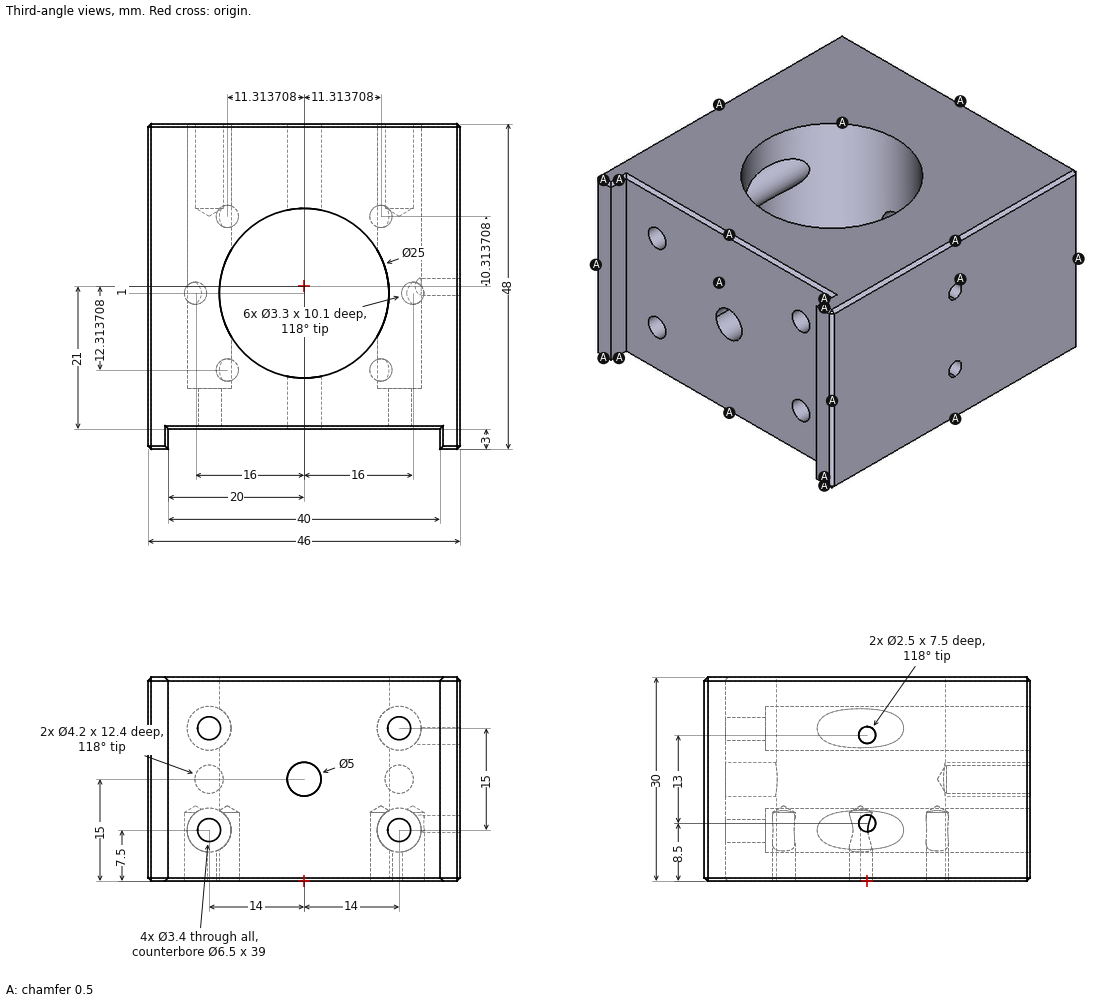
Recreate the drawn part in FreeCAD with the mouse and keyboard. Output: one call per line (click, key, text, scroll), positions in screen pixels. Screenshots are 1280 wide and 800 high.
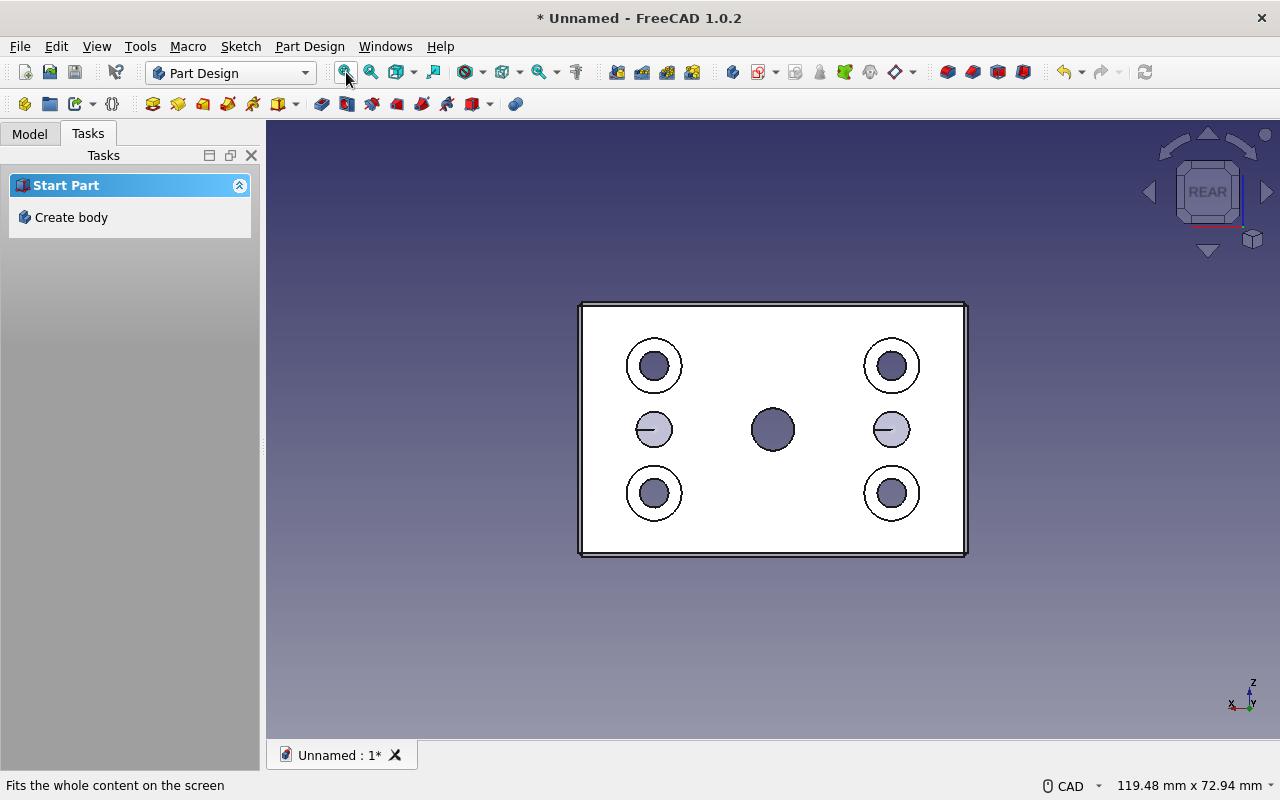
key(0)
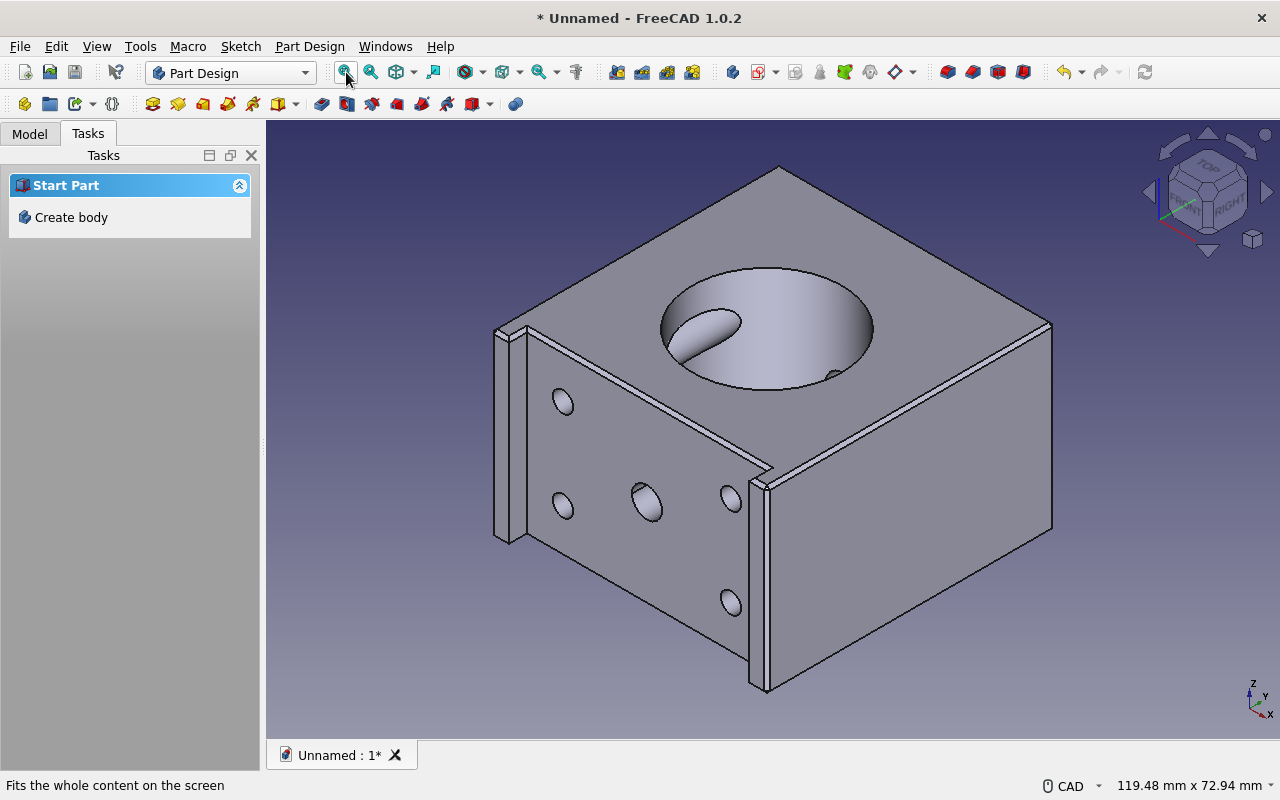
click(951, 485)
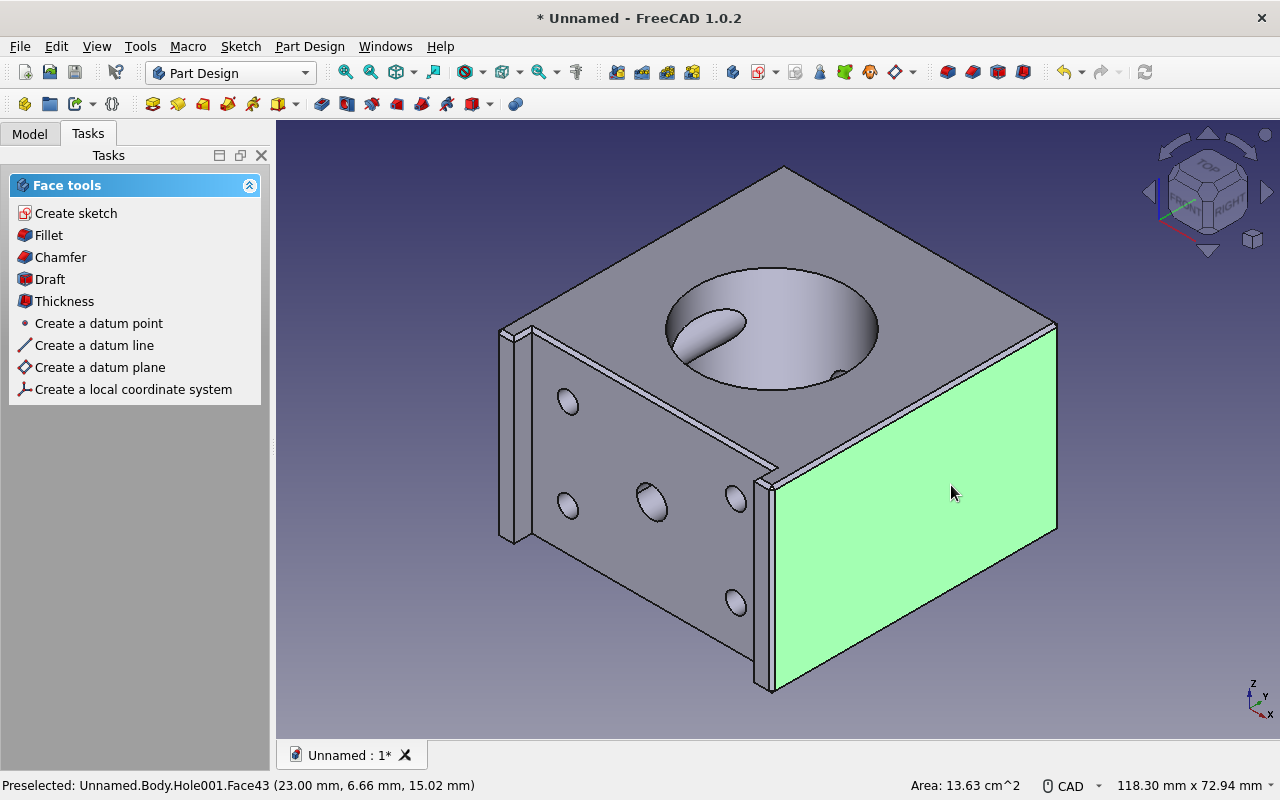
click(758, 72)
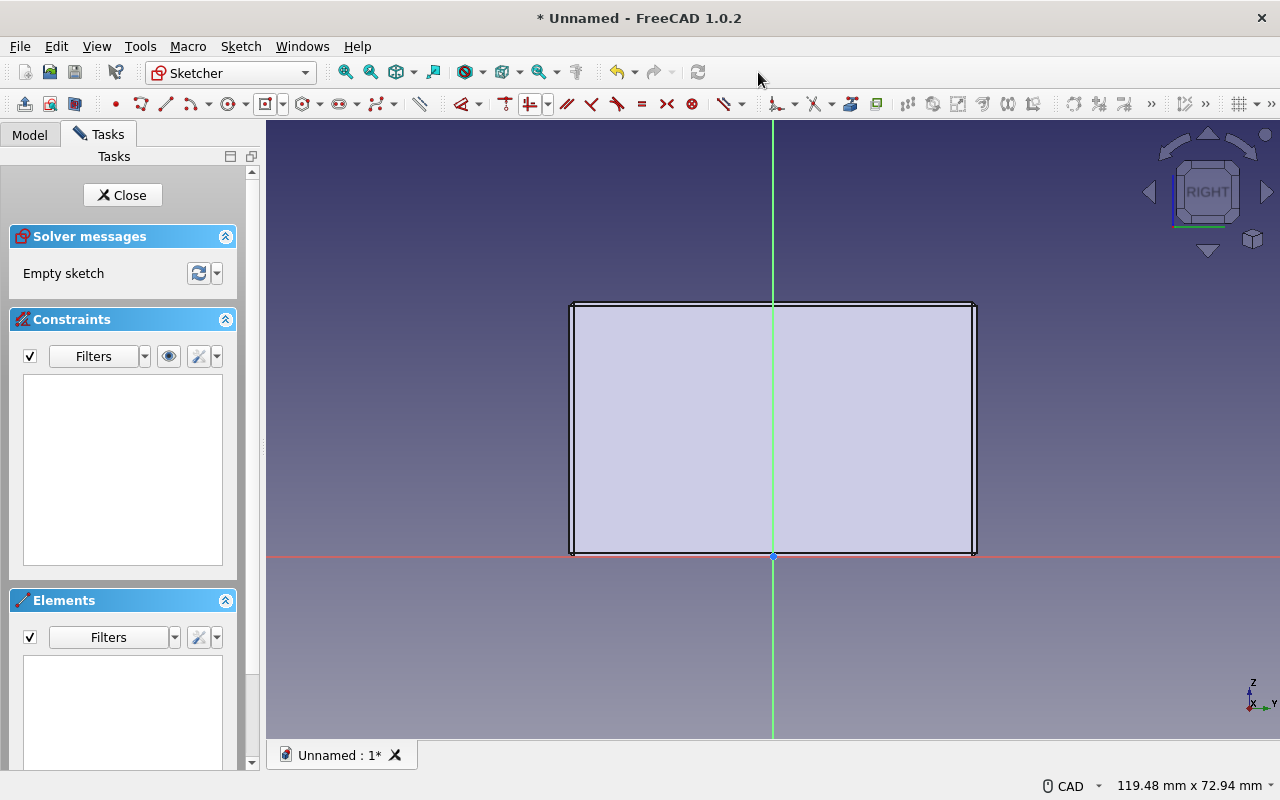
scroll(829, 485, up, 4)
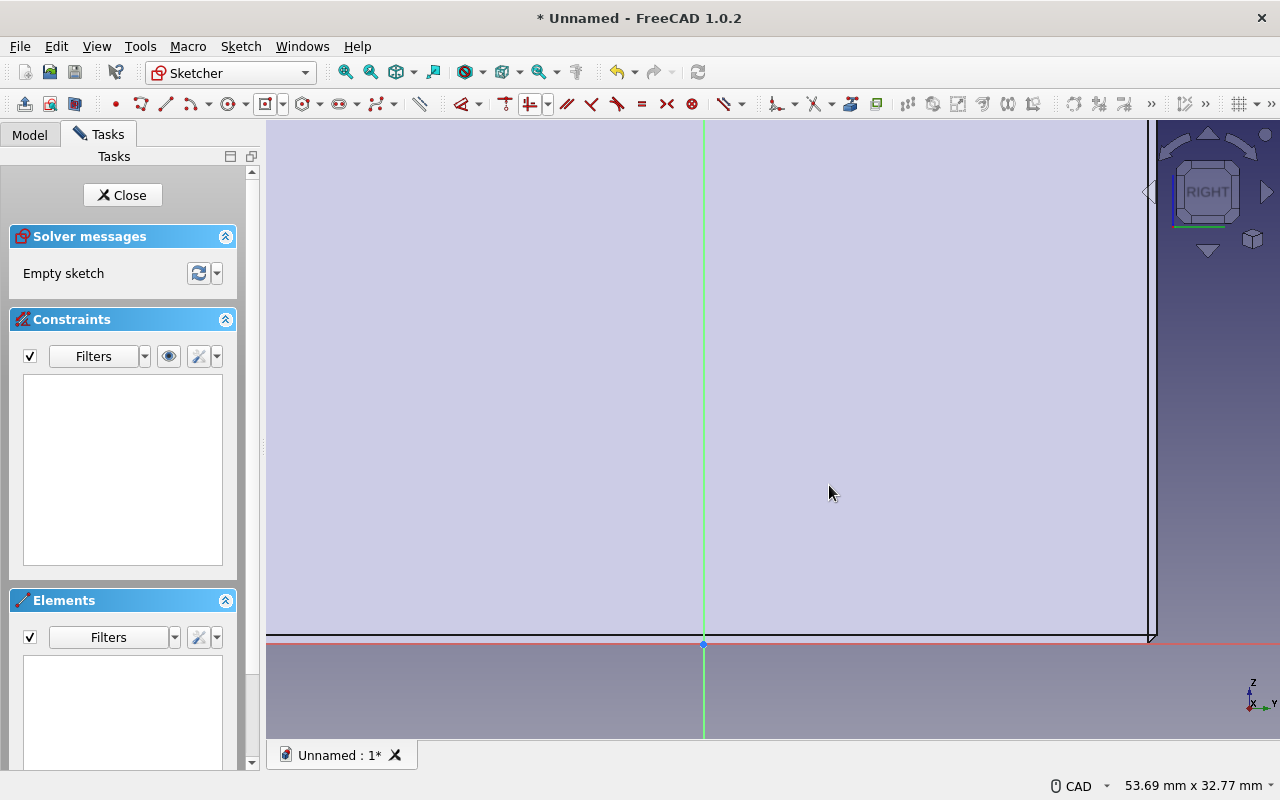
click(228, 104)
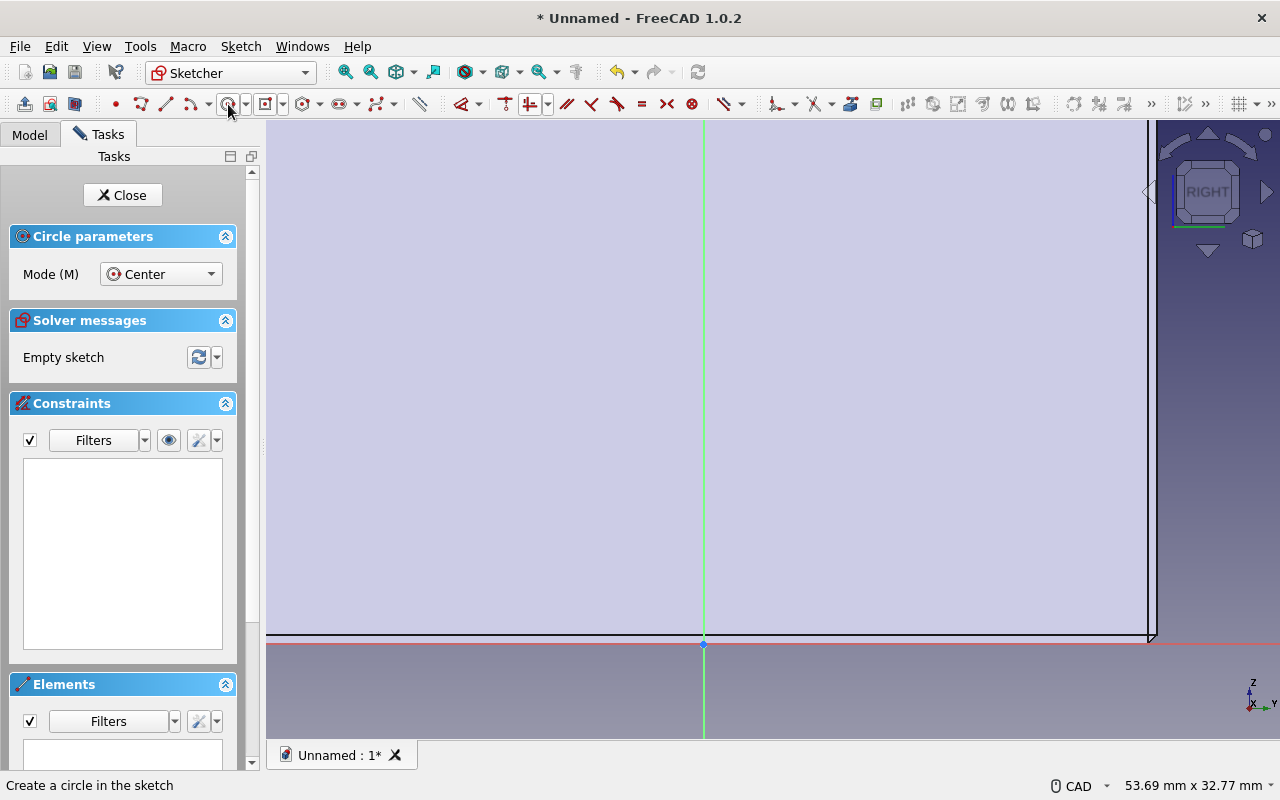
click(704, 238)
move(720, 221)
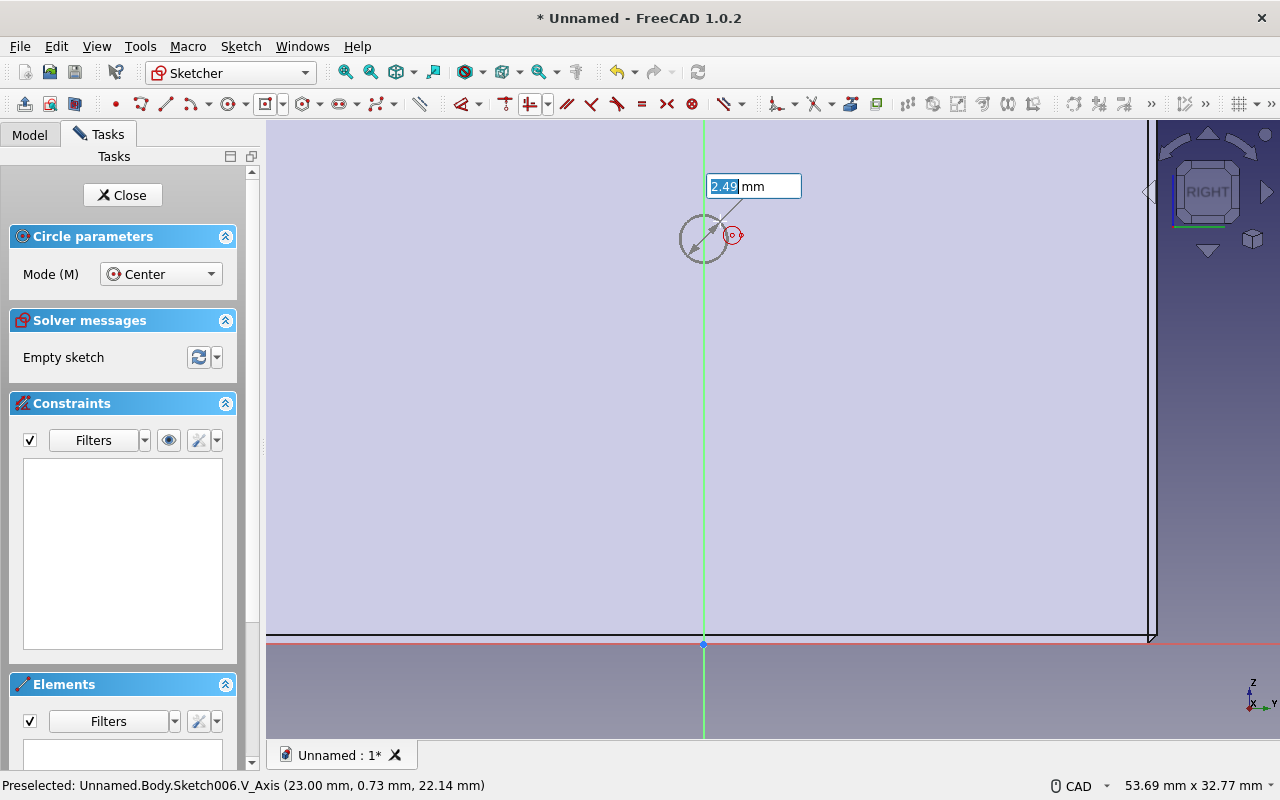
text(2.5)
key(Return)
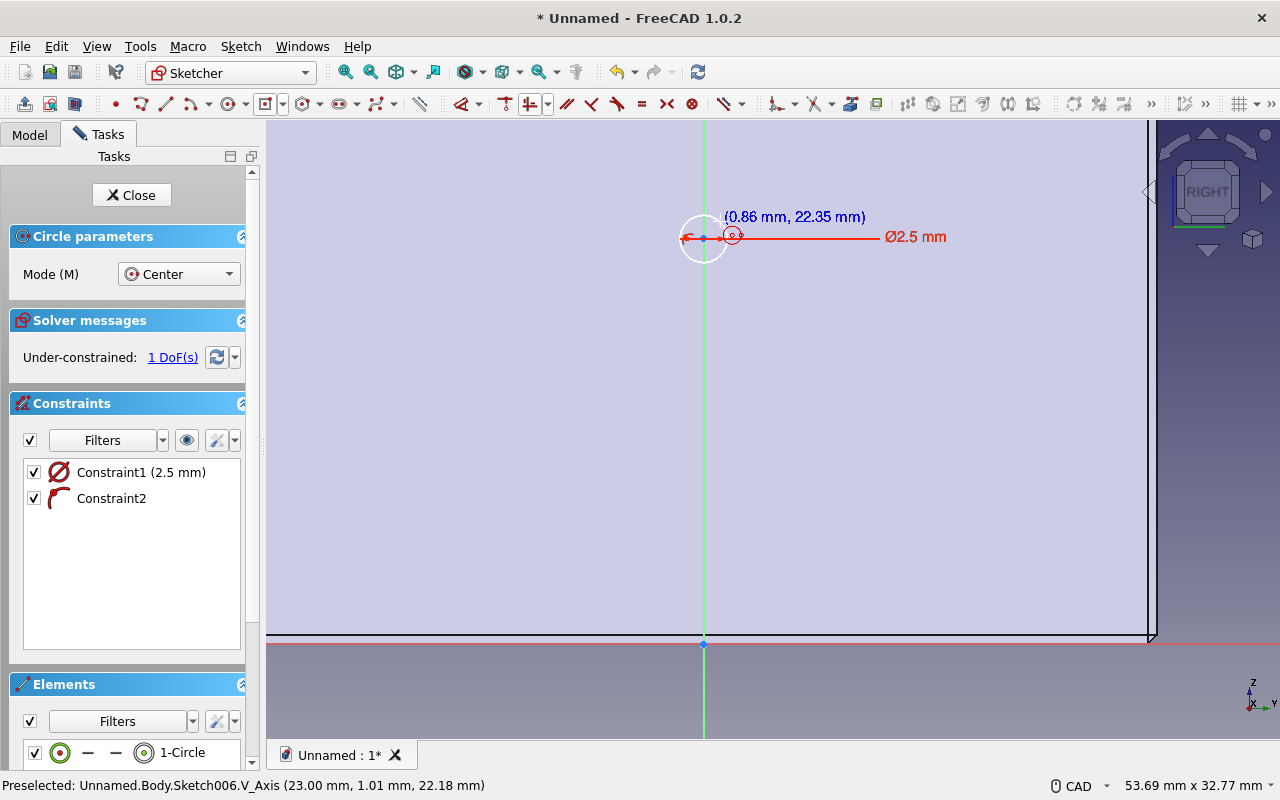
click(704, 484)
move(720, 467)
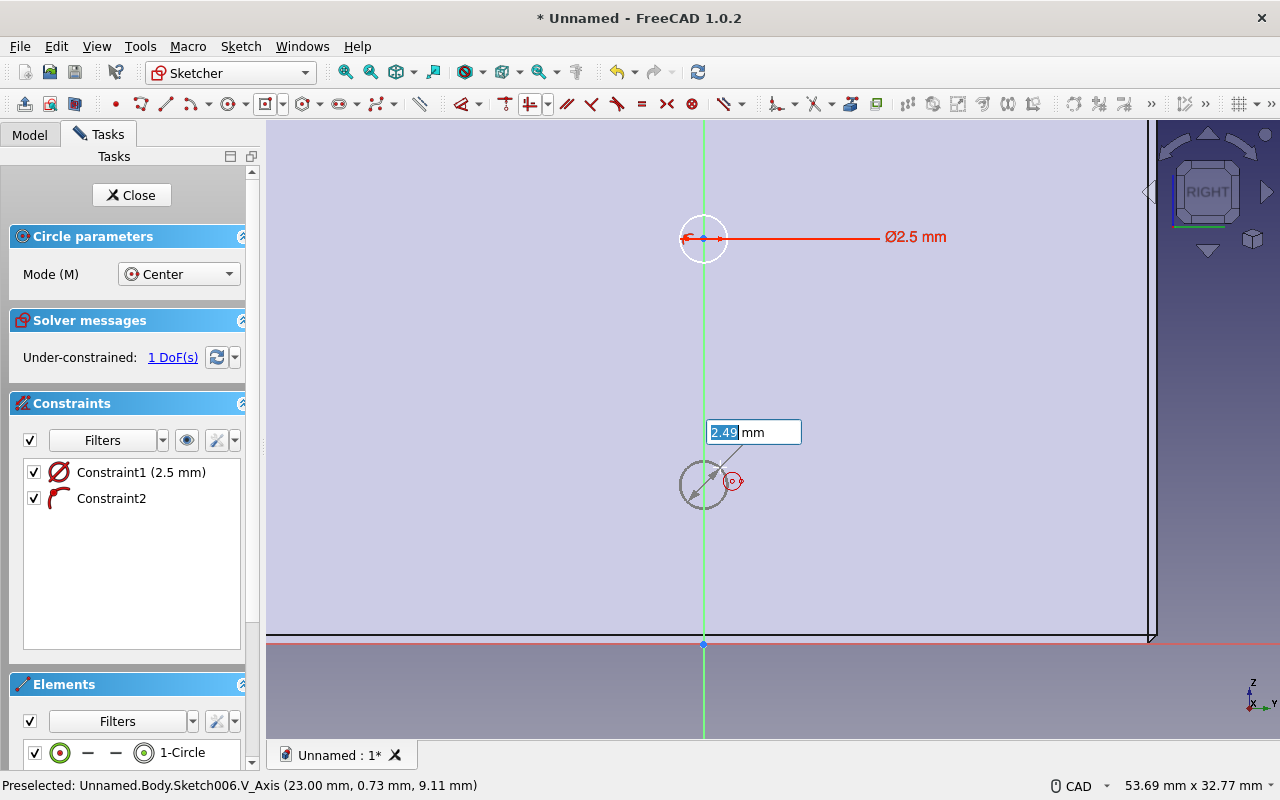
text(2.5)
key(Return)
key(Escape)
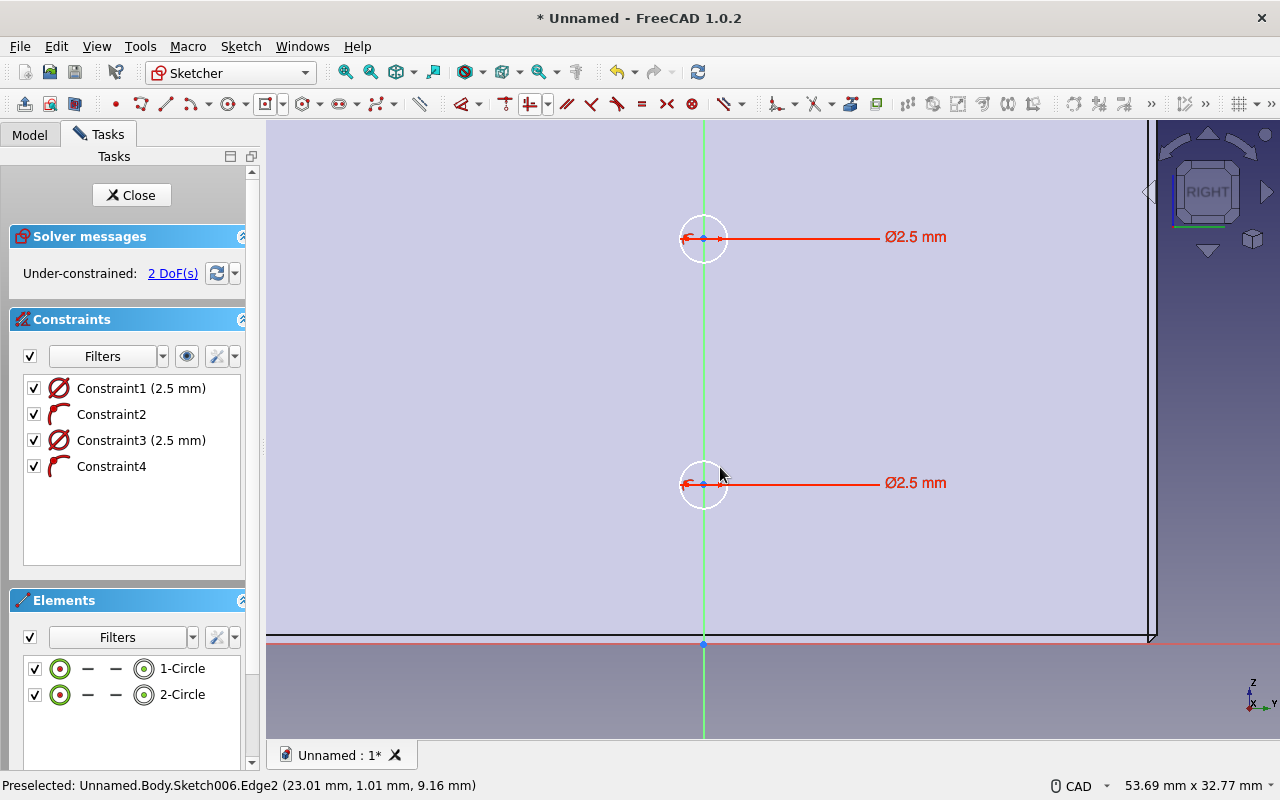
click(460, 104)